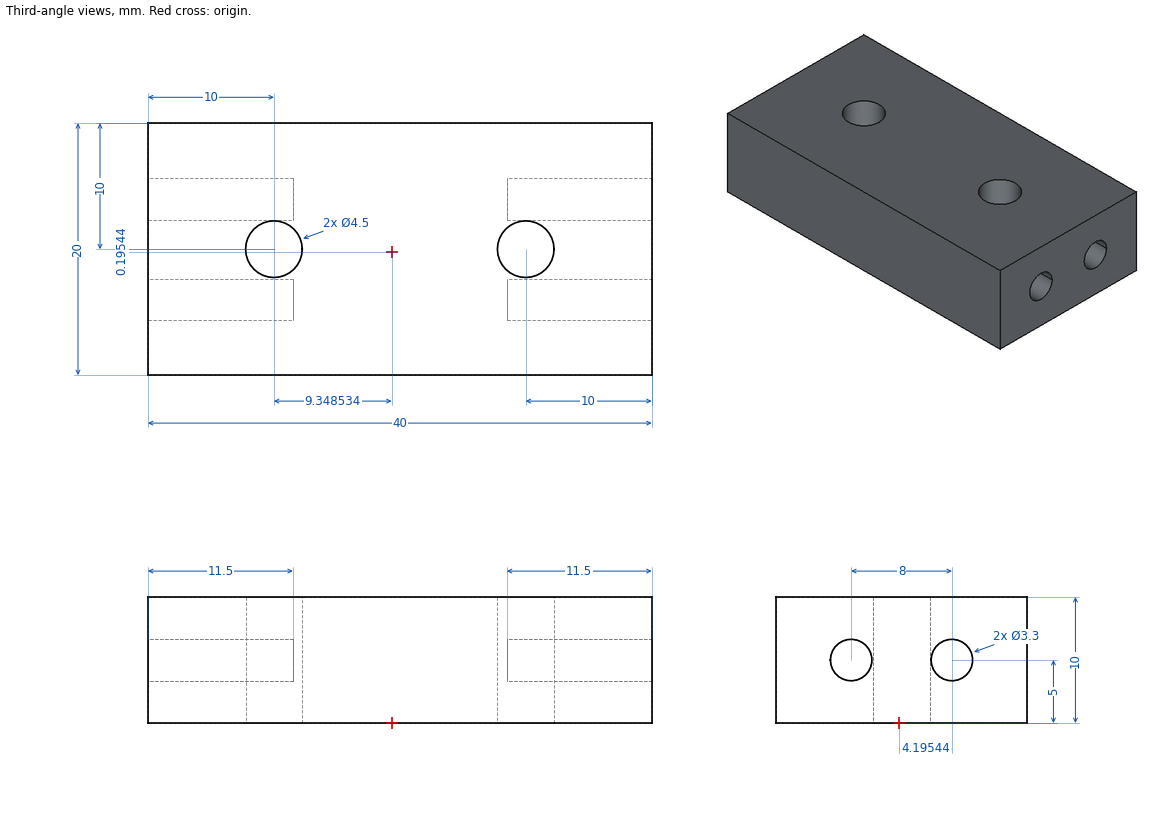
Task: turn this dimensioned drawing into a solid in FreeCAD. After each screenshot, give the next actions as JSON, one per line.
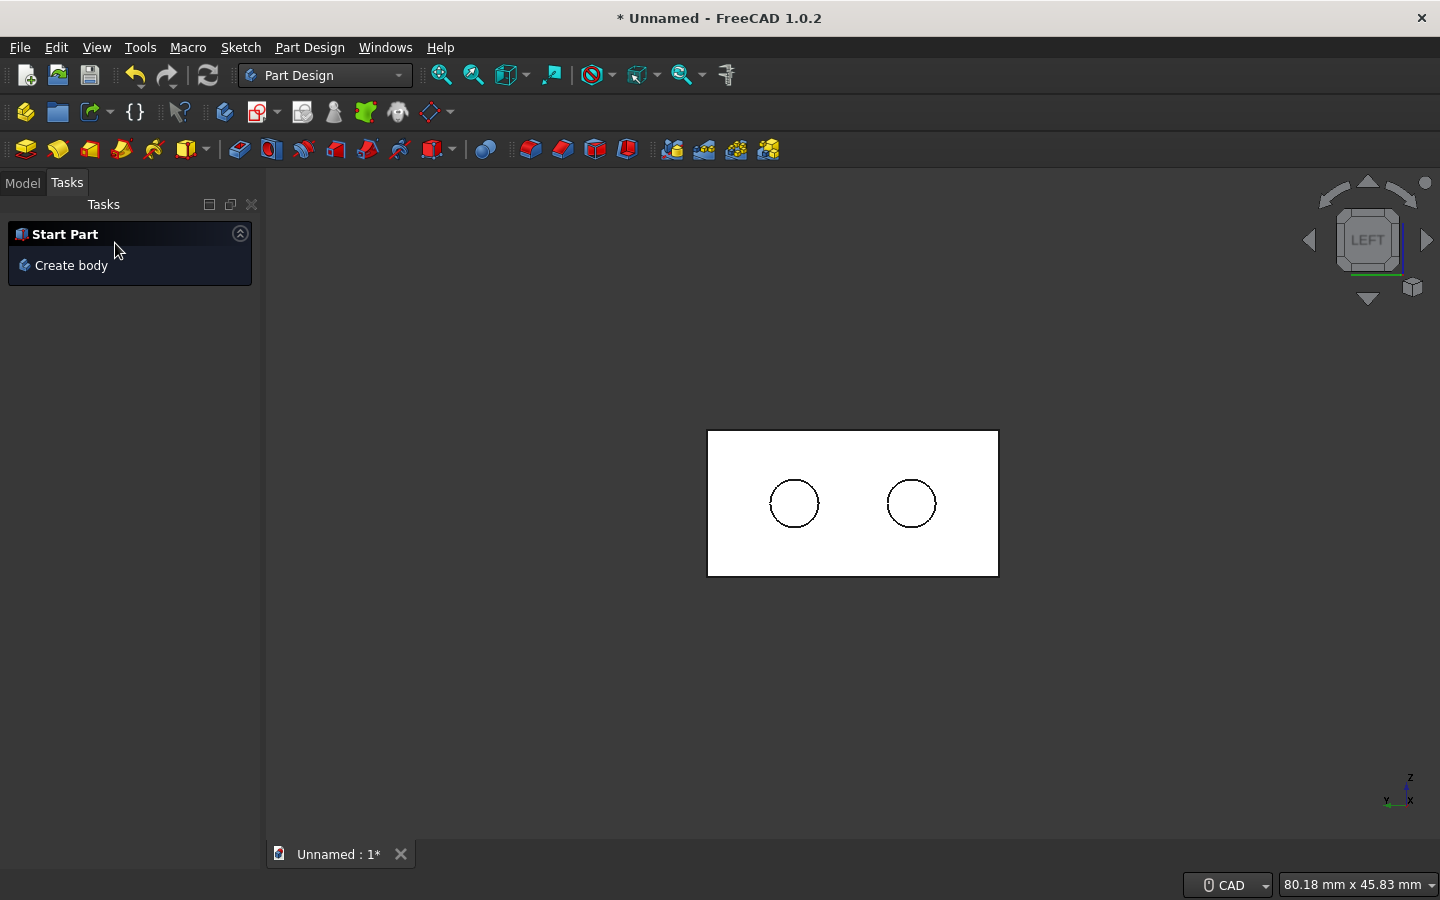
{"action": "left_click", "coordinate": [442, 76]}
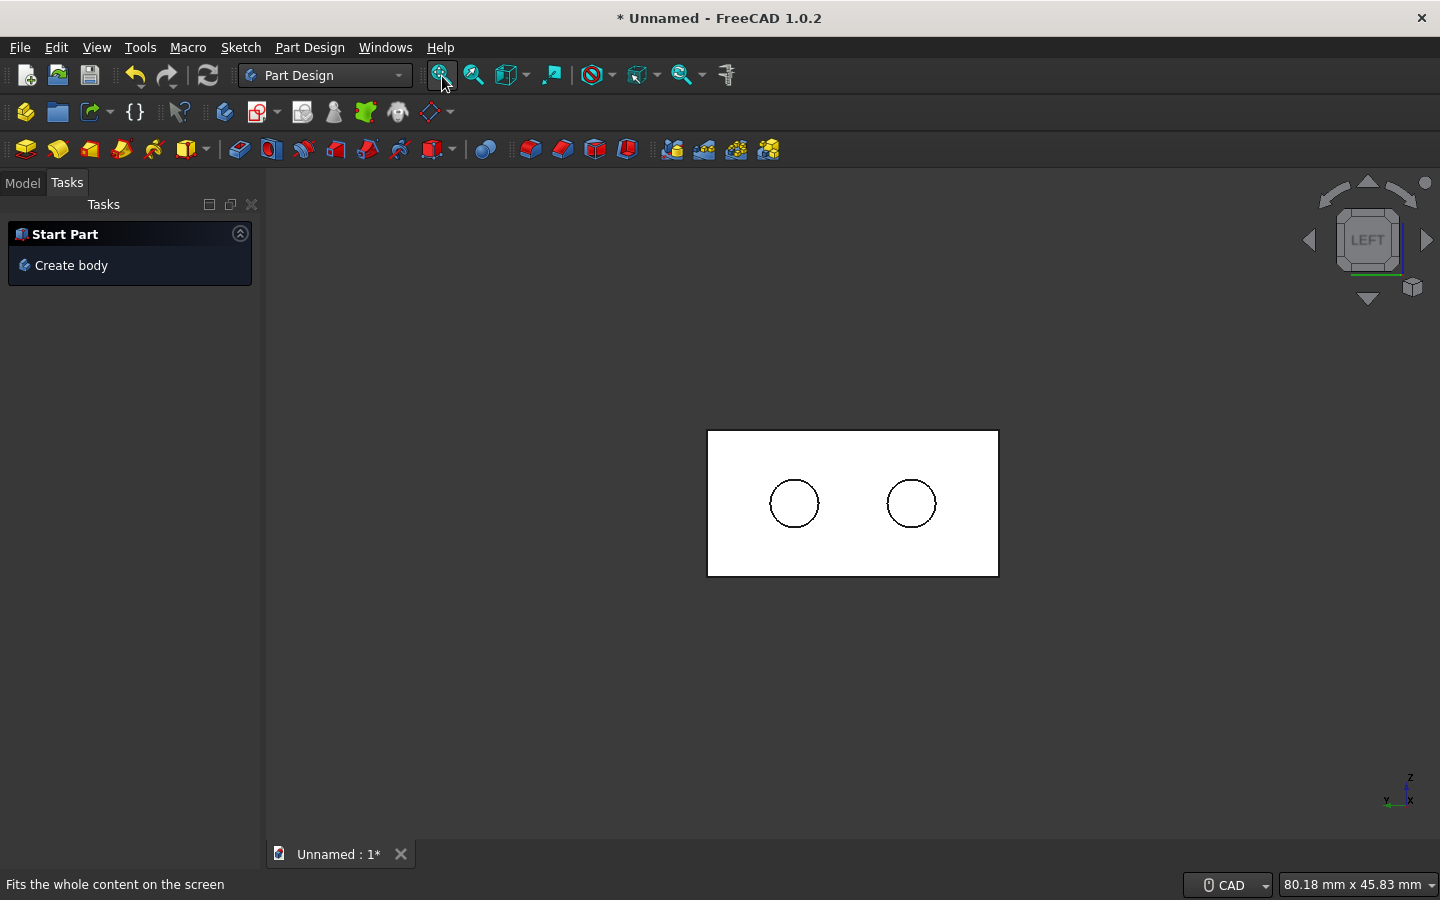
{"action": "left_click", "coordinate": [23, 182]}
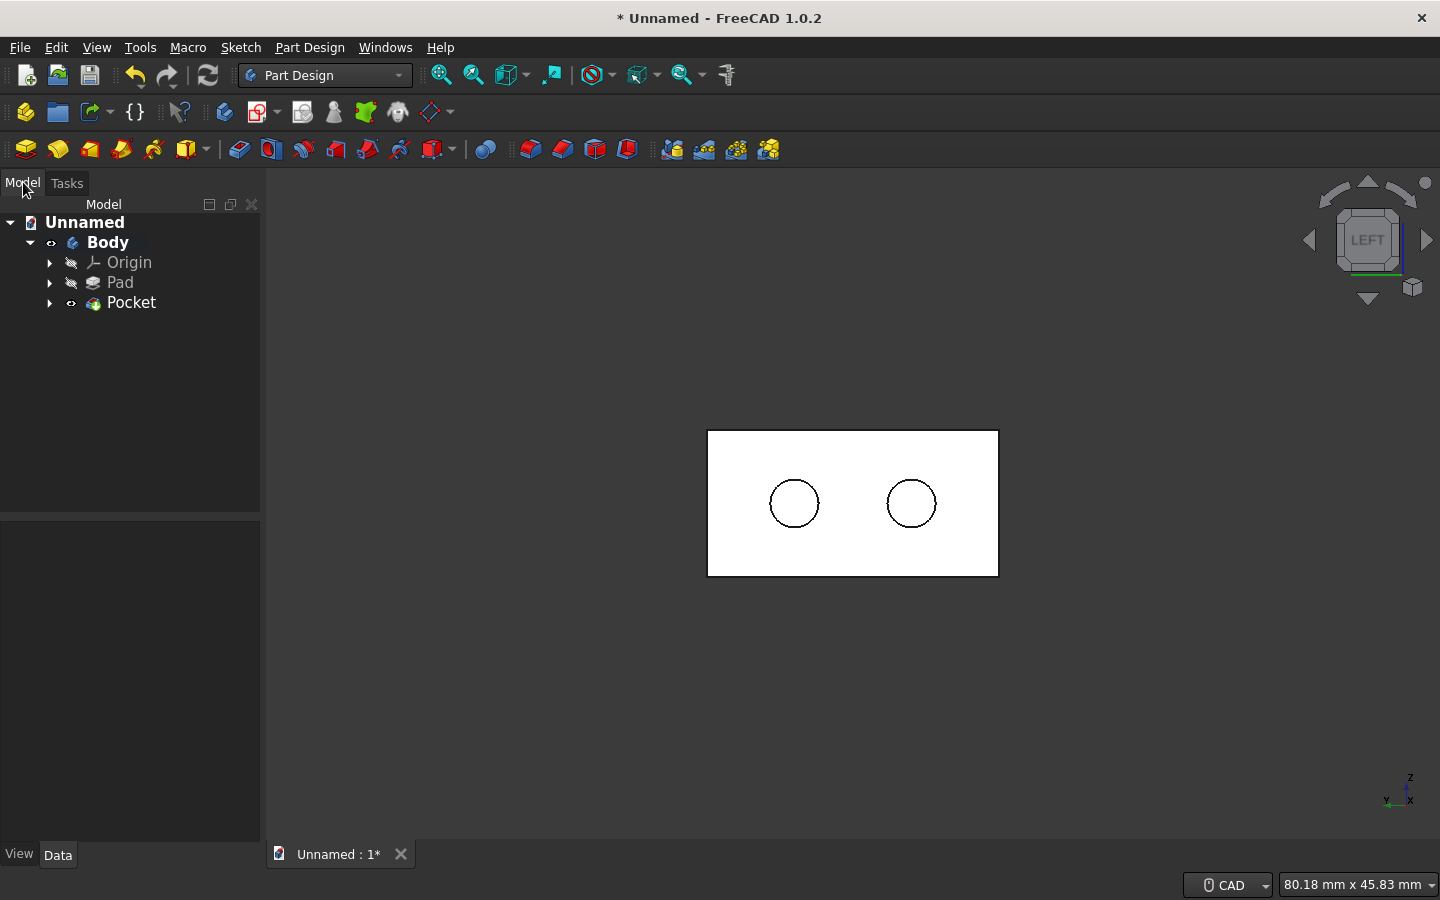
{"action": "left_click", "coordinate": [50, 263]}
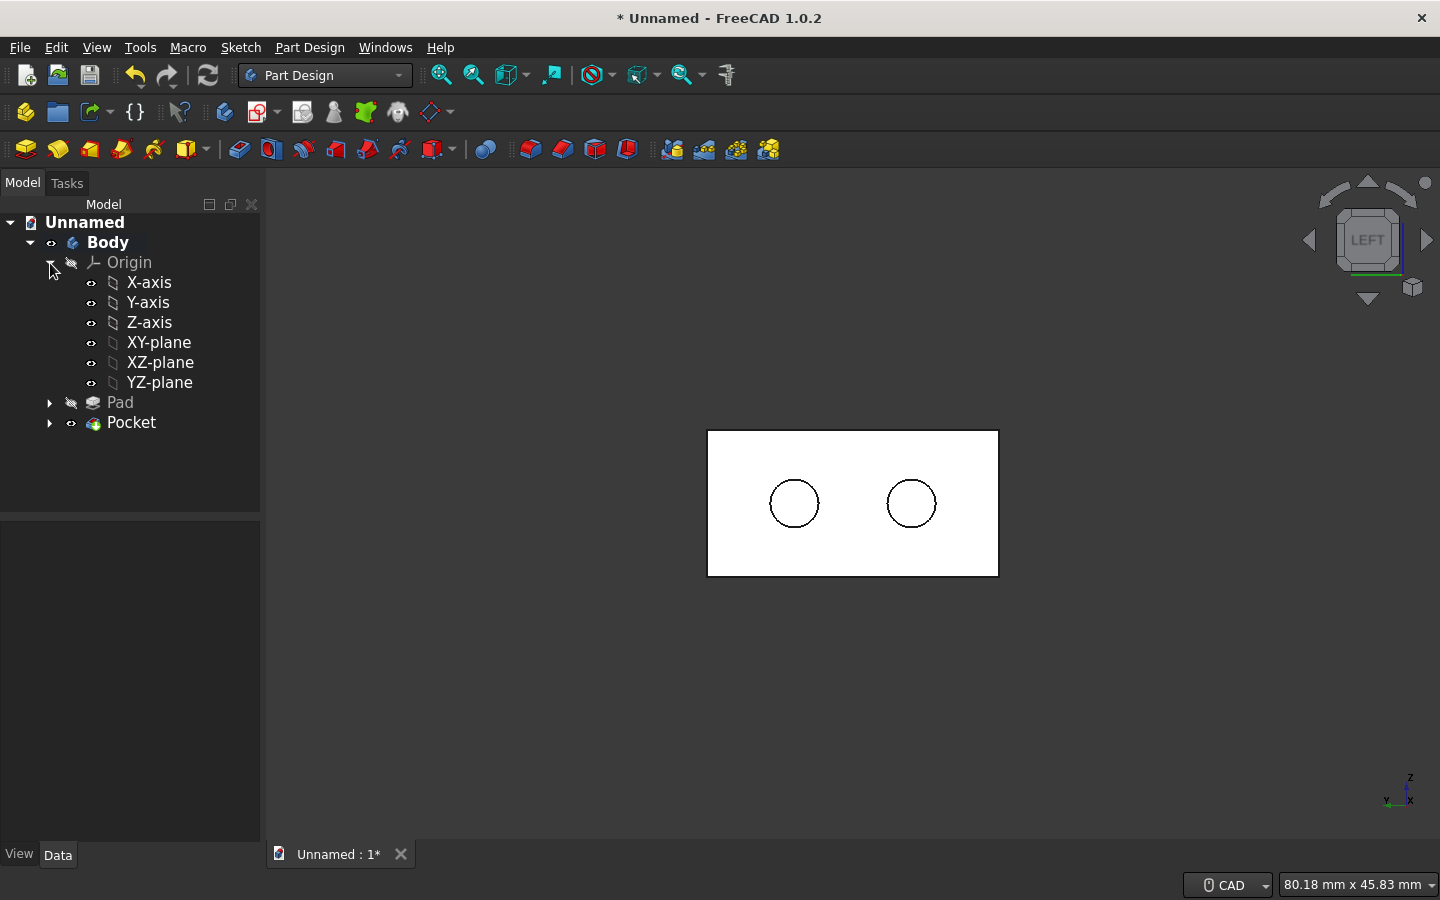
{"action": "left_click", "coordinate": [136, 383]}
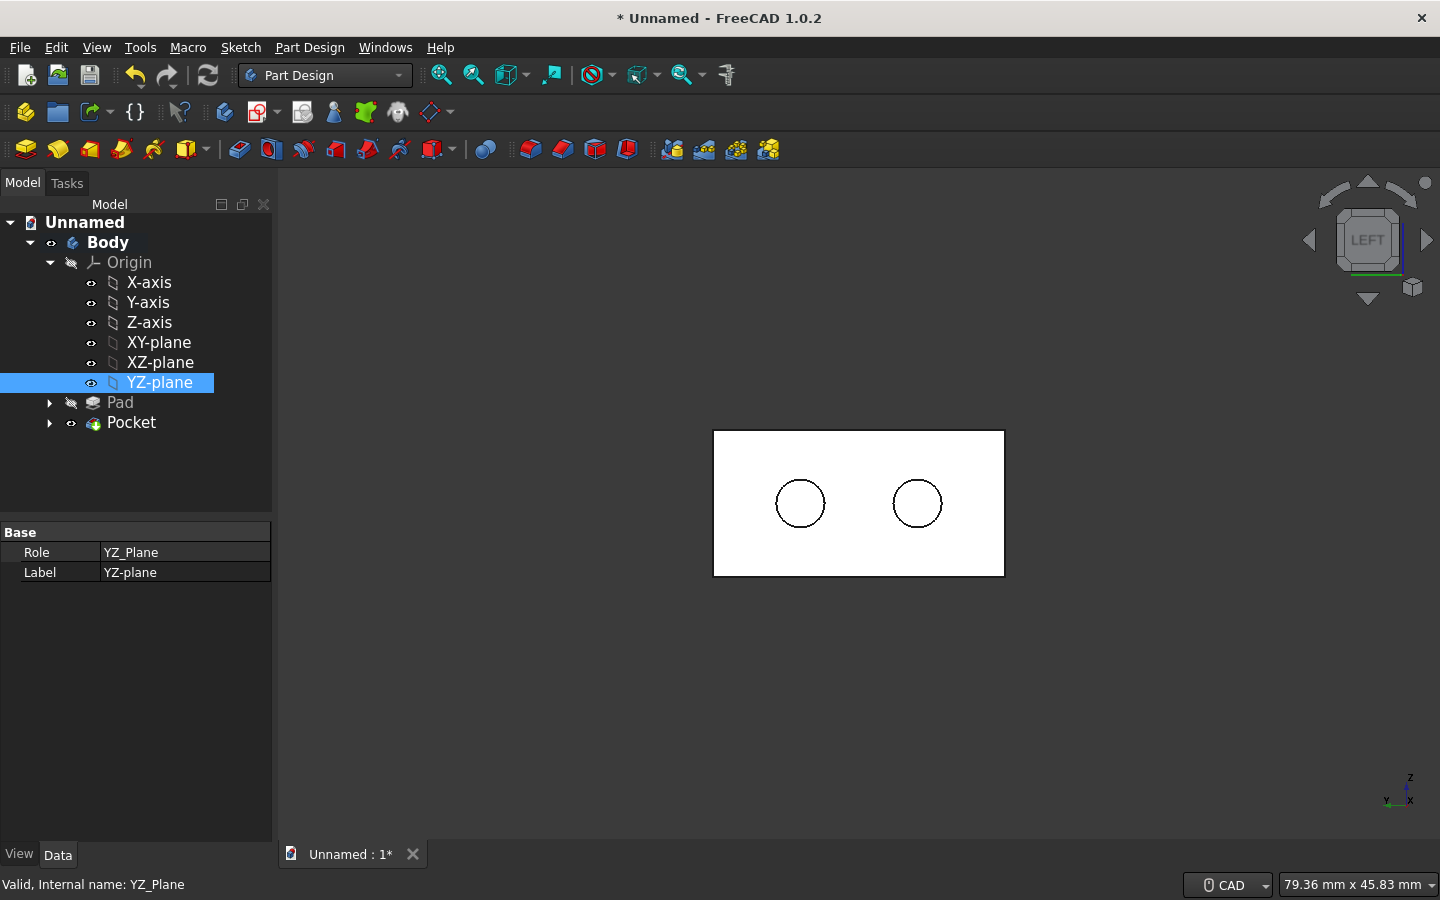
{"action": "left_click", "coordinate": [430, 112]}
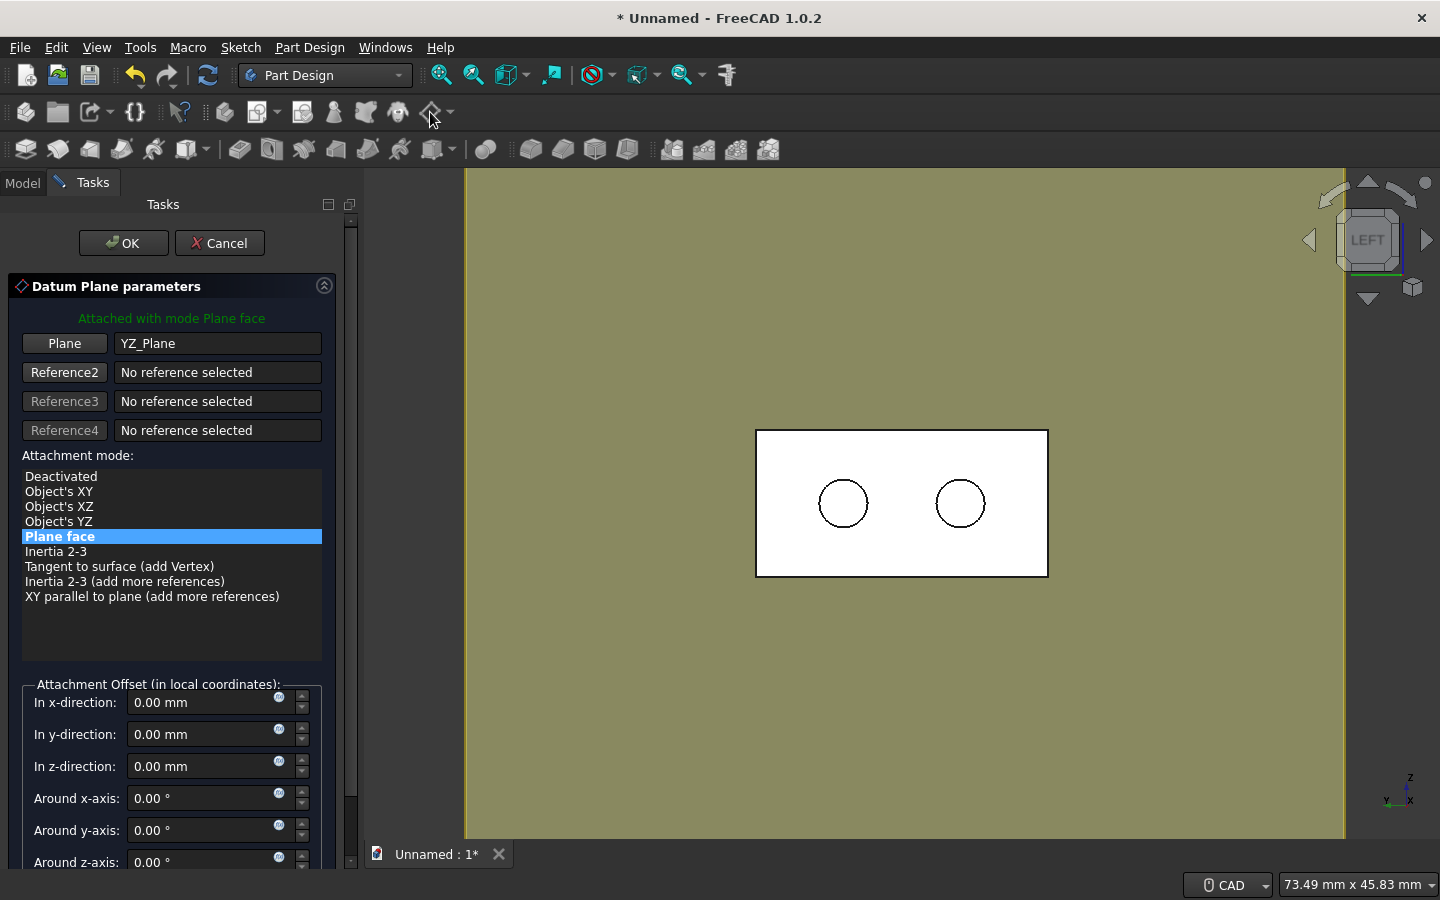
{"action": "triple_click", "coordinate": [210, 766]}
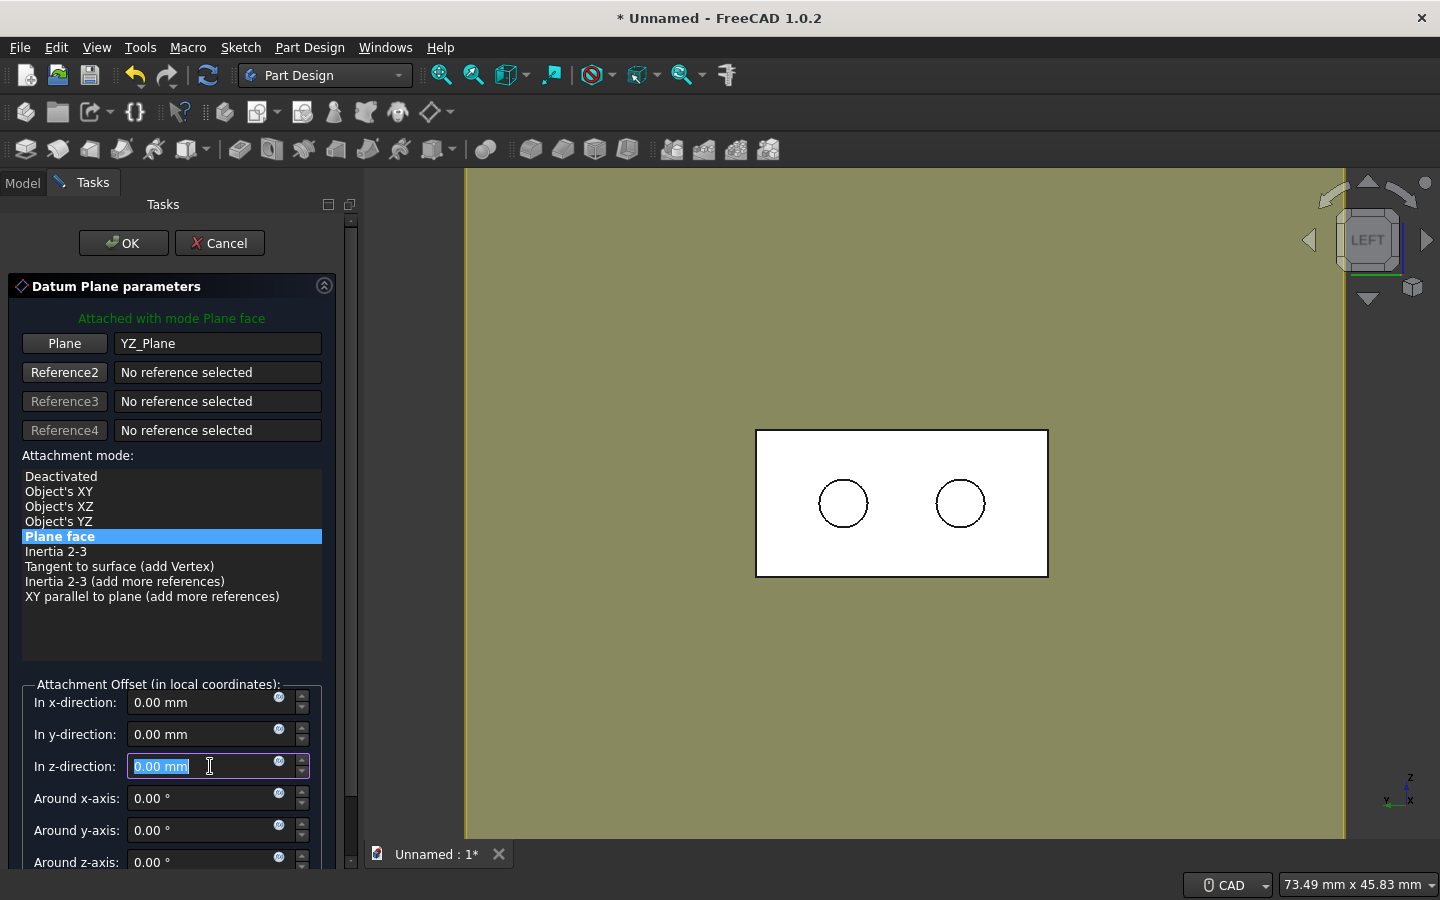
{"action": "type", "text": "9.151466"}
{"action": "key", "text": "Tab"}